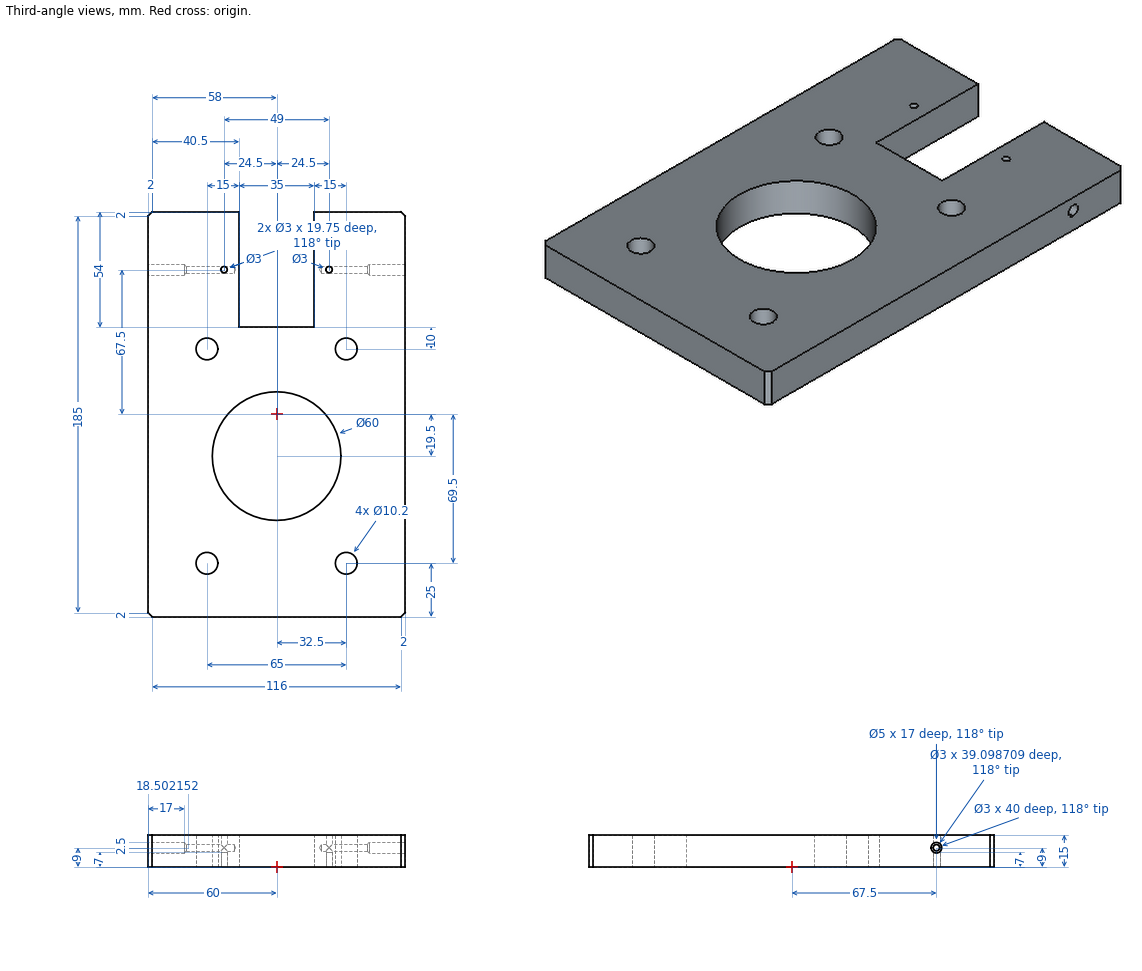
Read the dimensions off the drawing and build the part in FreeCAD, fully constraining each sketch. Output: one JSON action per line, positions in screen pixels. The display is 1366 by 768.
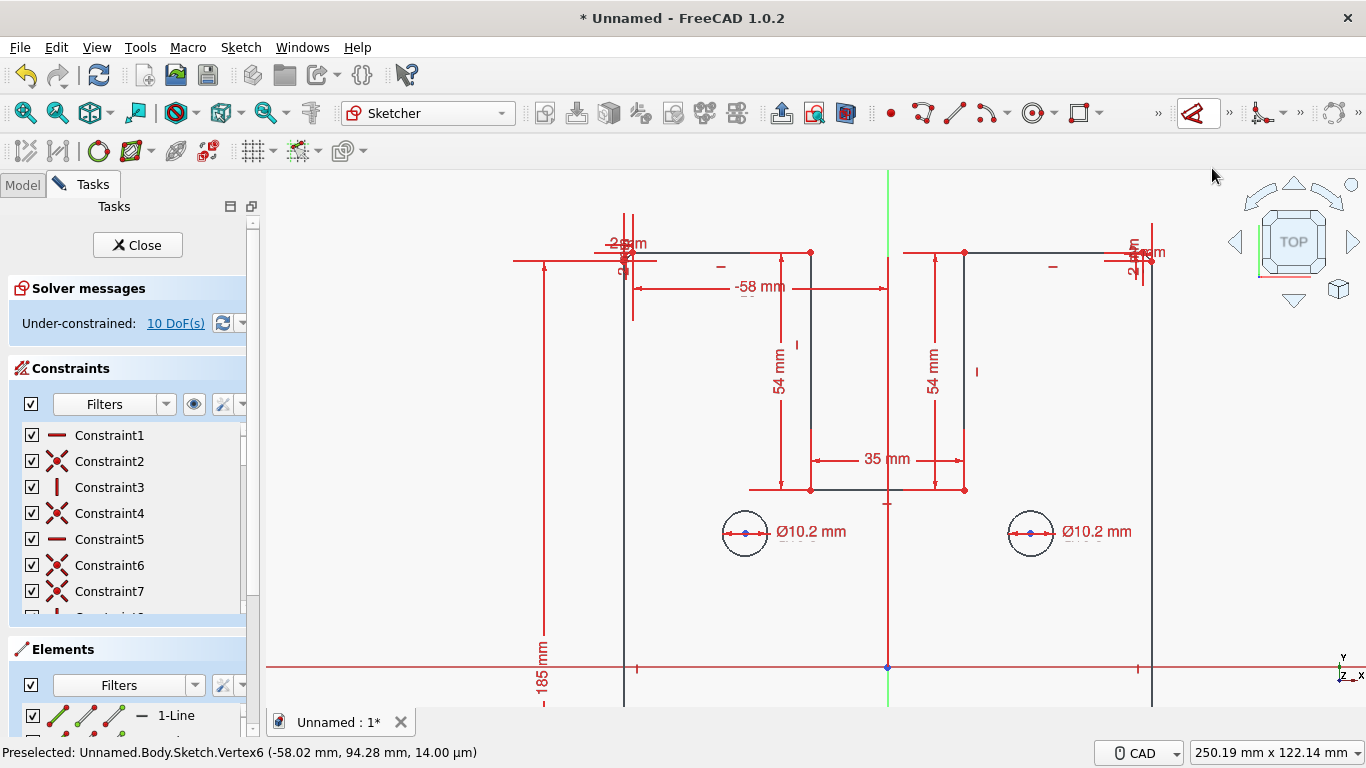
{"action": "scroll", "coordinate": [633, 252], "scroll_direction": "down", "scroll_amount": 4}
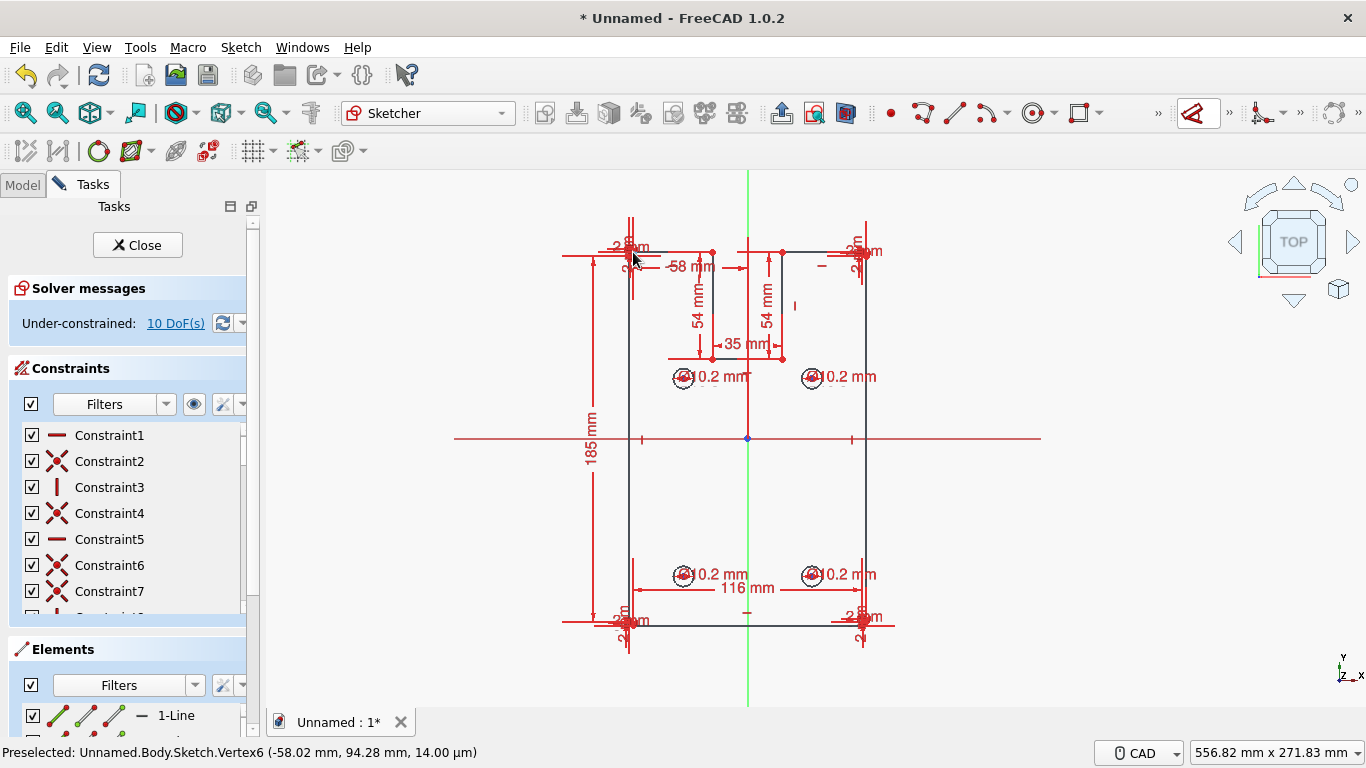
{"action": "scroll", "coordinate": [862, 626], "scroll_direction": "up", "scroll_amount": 4}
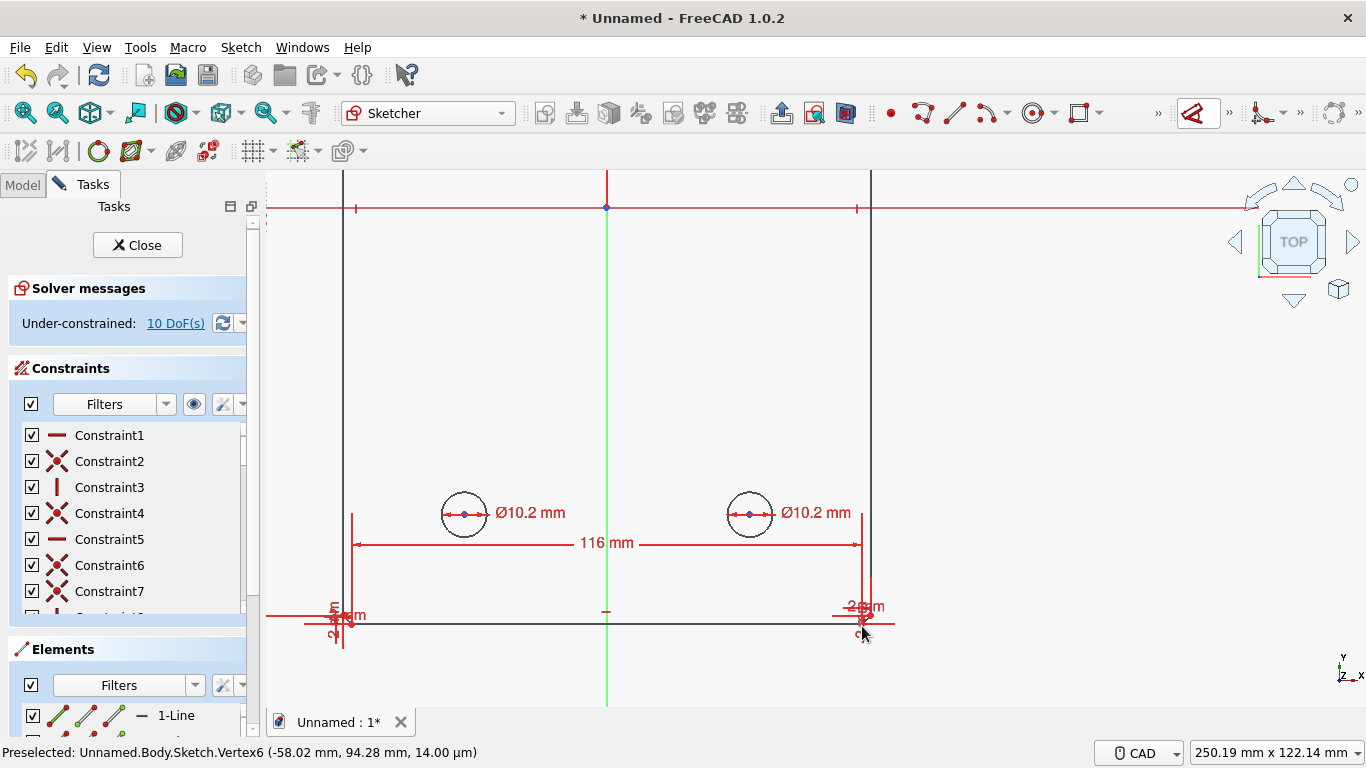
{"action": "left_click", "coordinate": [862, 624]}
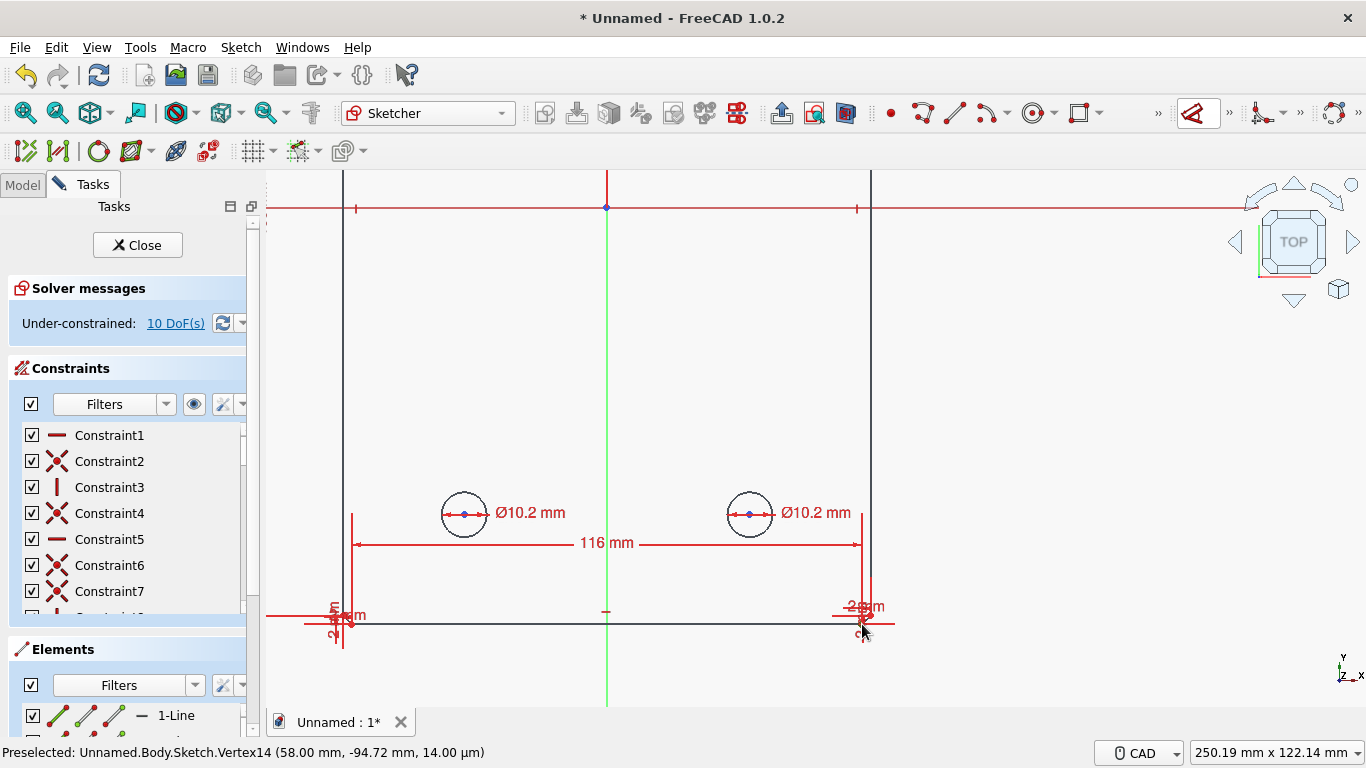
{"action": "left_click", "coordinate": [750, 515]}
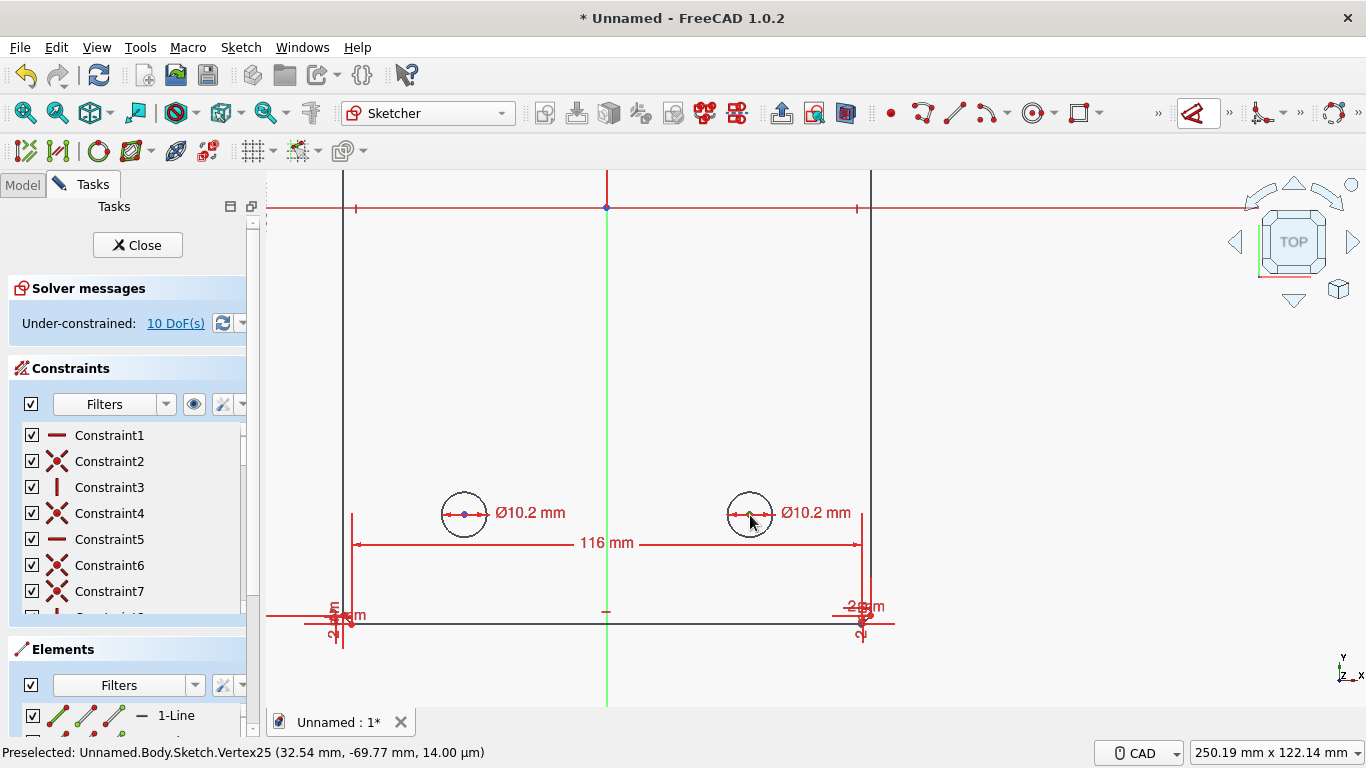
{"action": "key", "text": "i"}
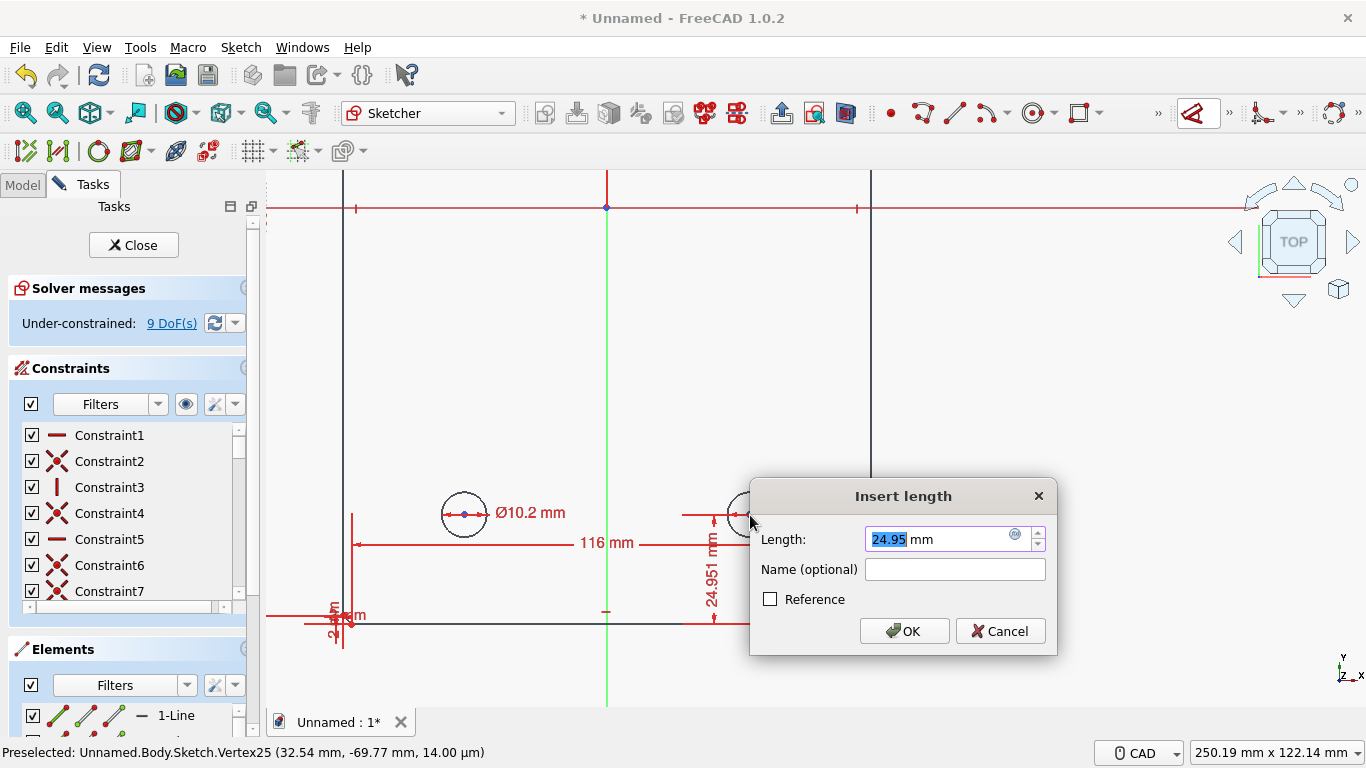
{"action": "type", "text": "25"}
{"action": "key", "text": "Return"}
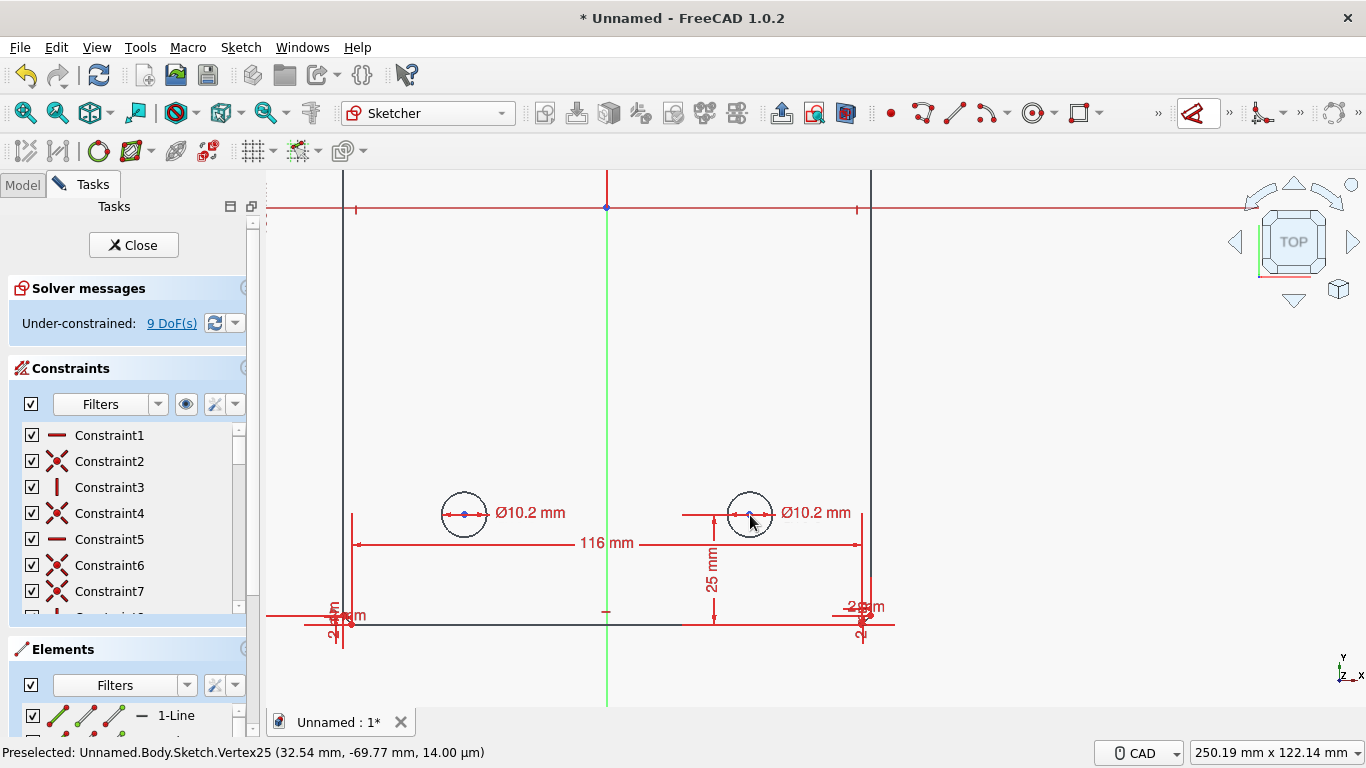
{"action": "left_click", "coordinate": [750, 515]}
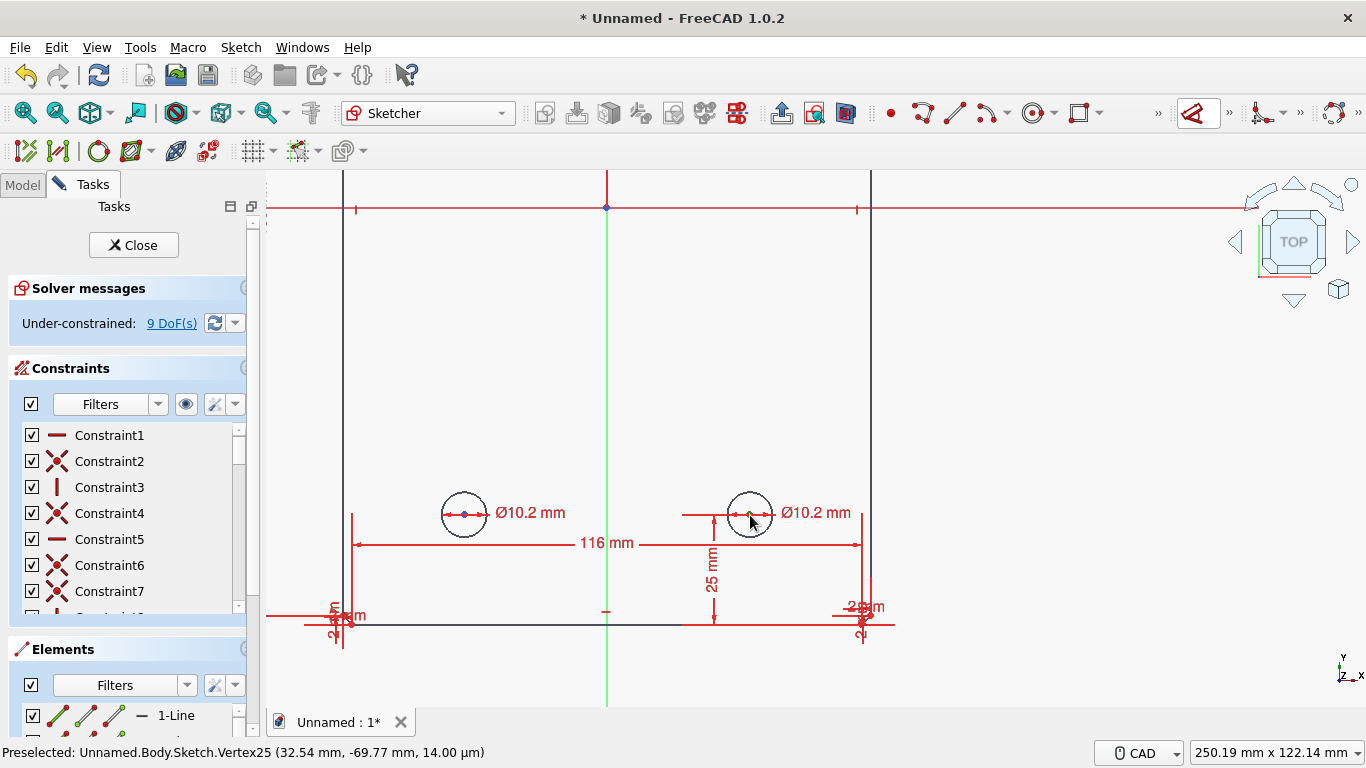
{"action": "left_click", "coordinate": [464, 515]}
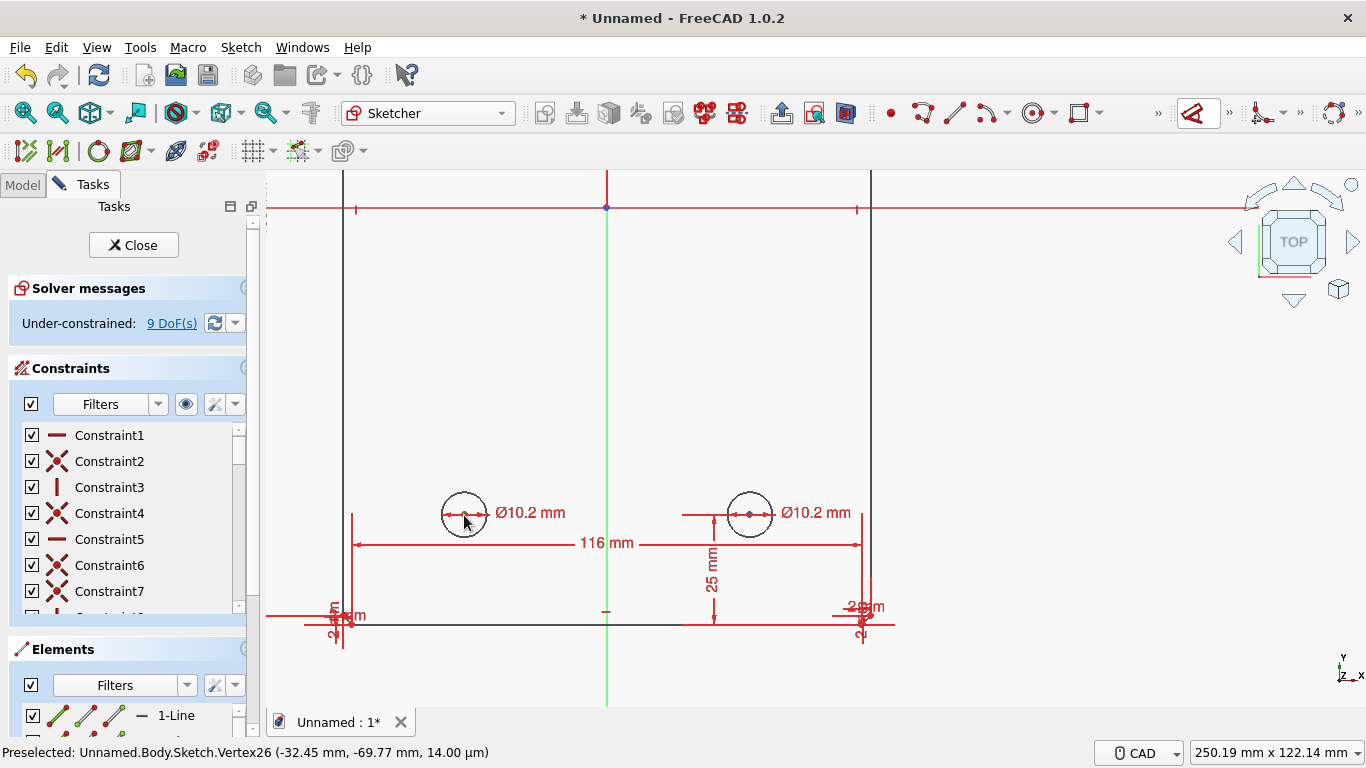
{"action": "key", "text": "l"}